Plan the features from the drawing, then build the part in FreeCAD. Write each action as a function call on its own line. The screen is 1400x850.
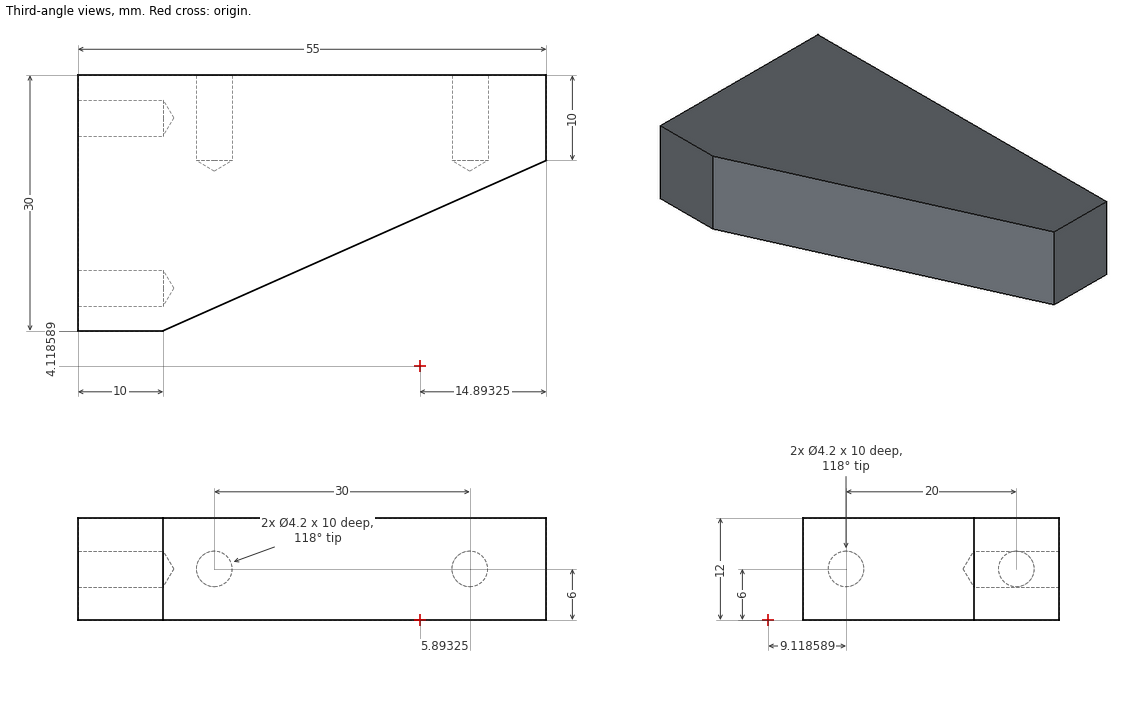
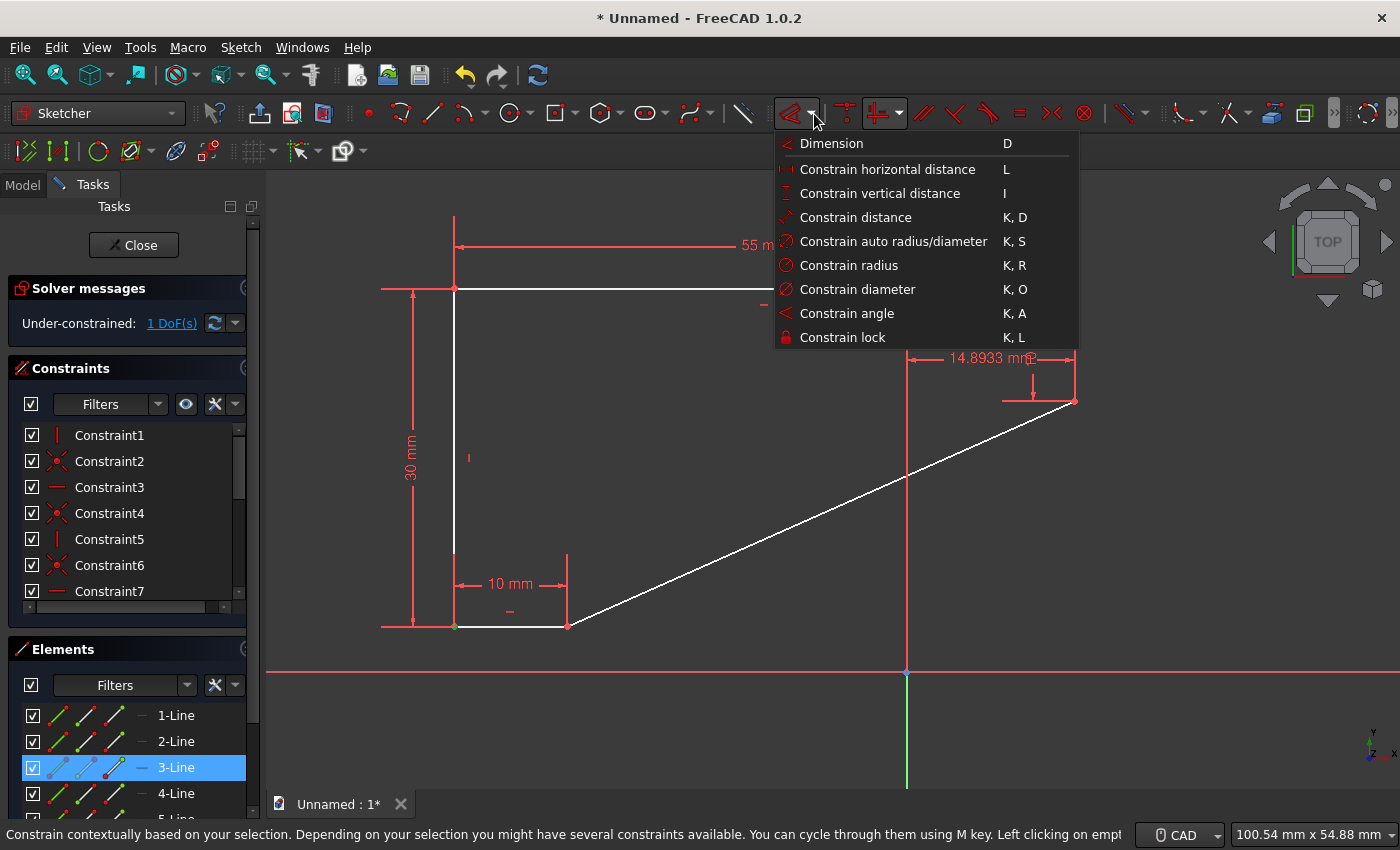
click(927, 193)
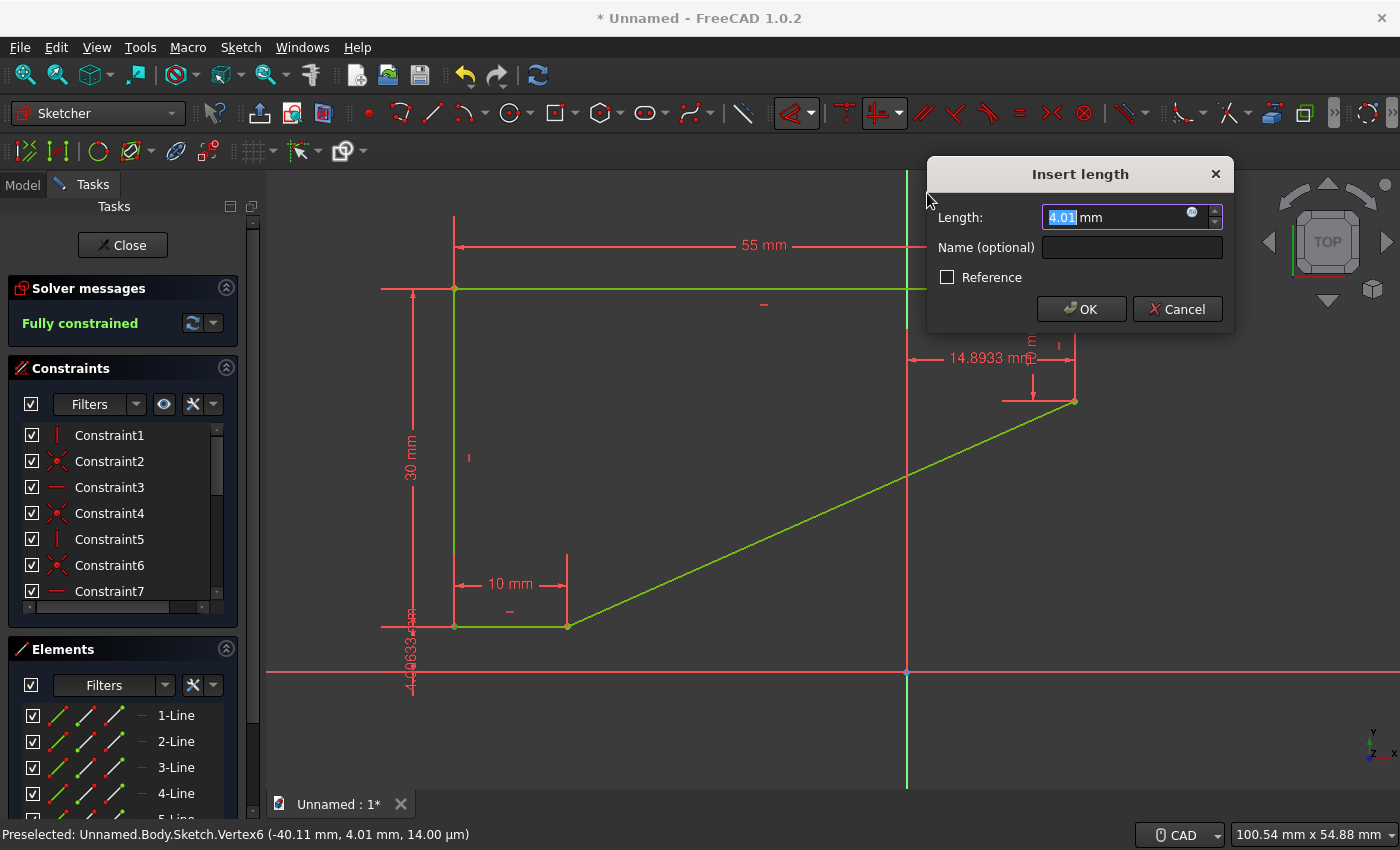
text(4.118589)
key(Return)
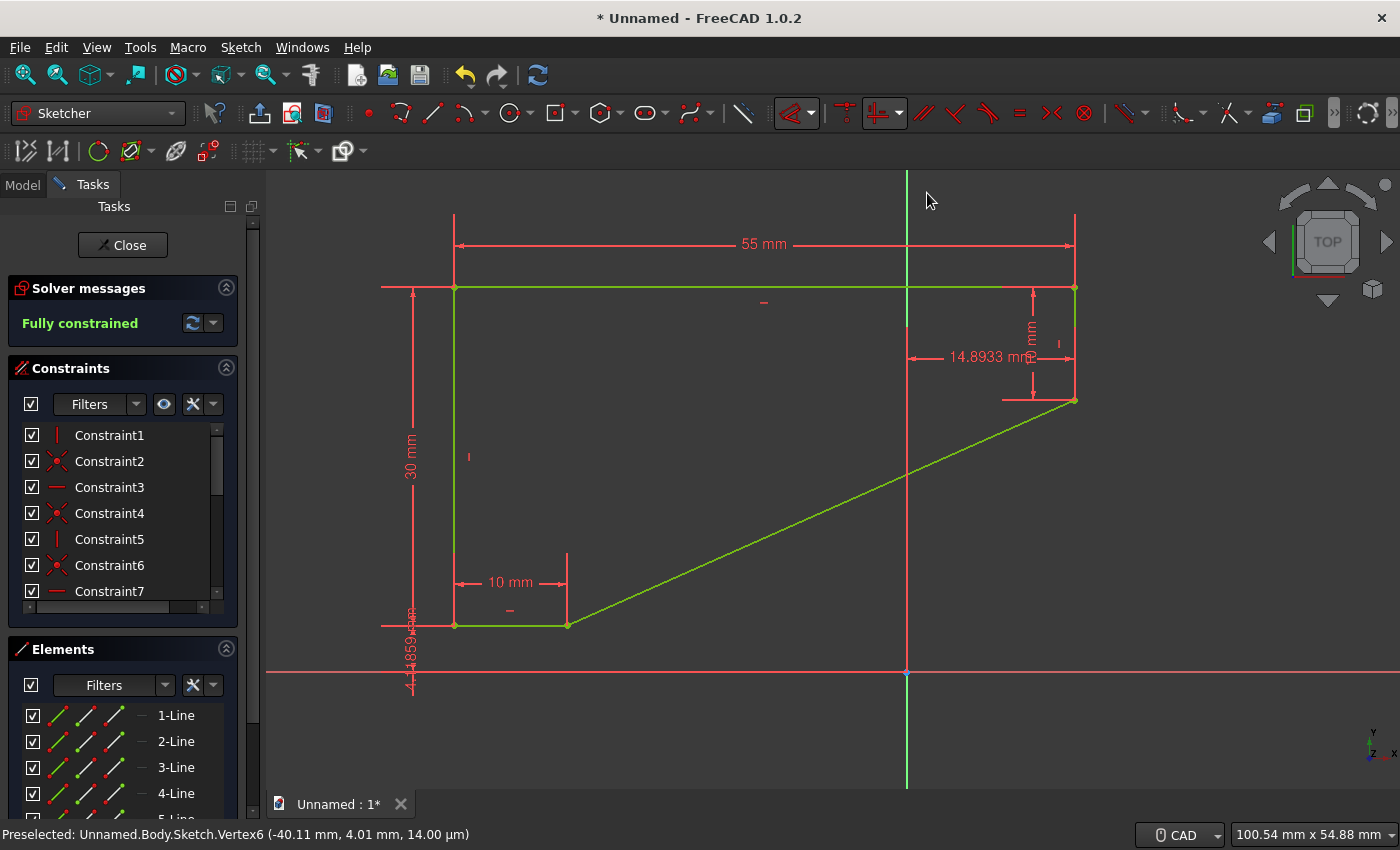
click(123, 245)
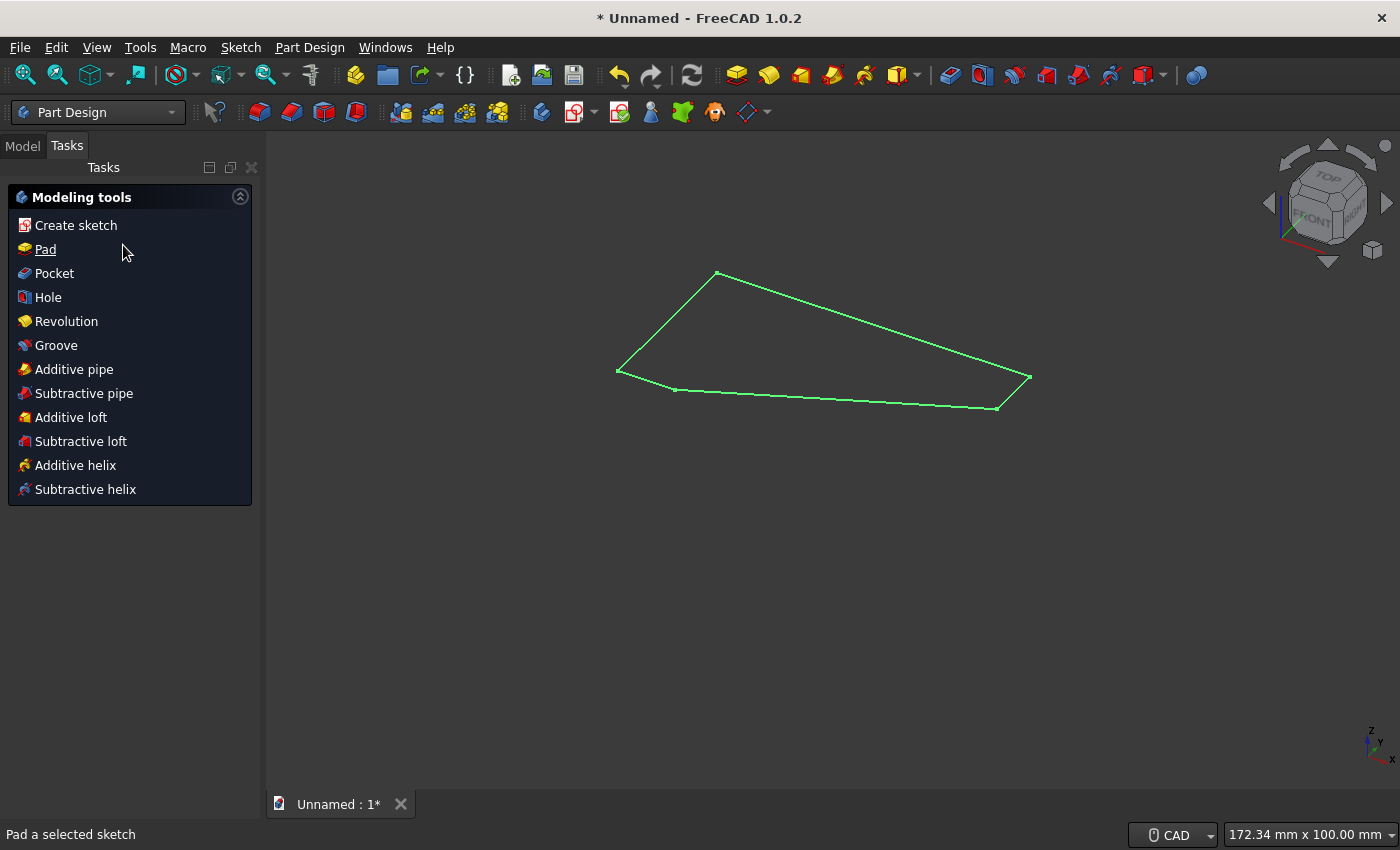
click(738, 76)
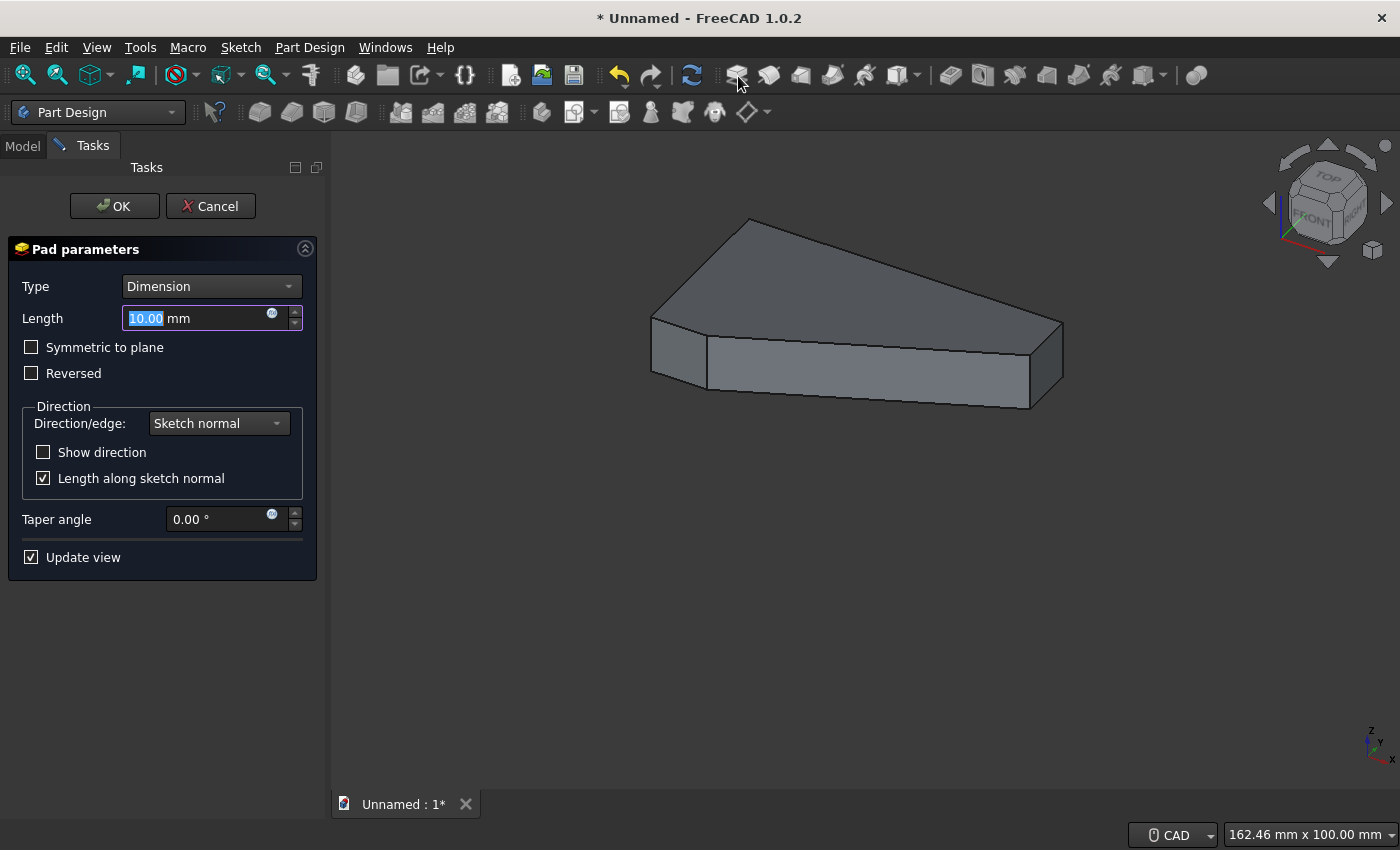
text(12)
key(Tab)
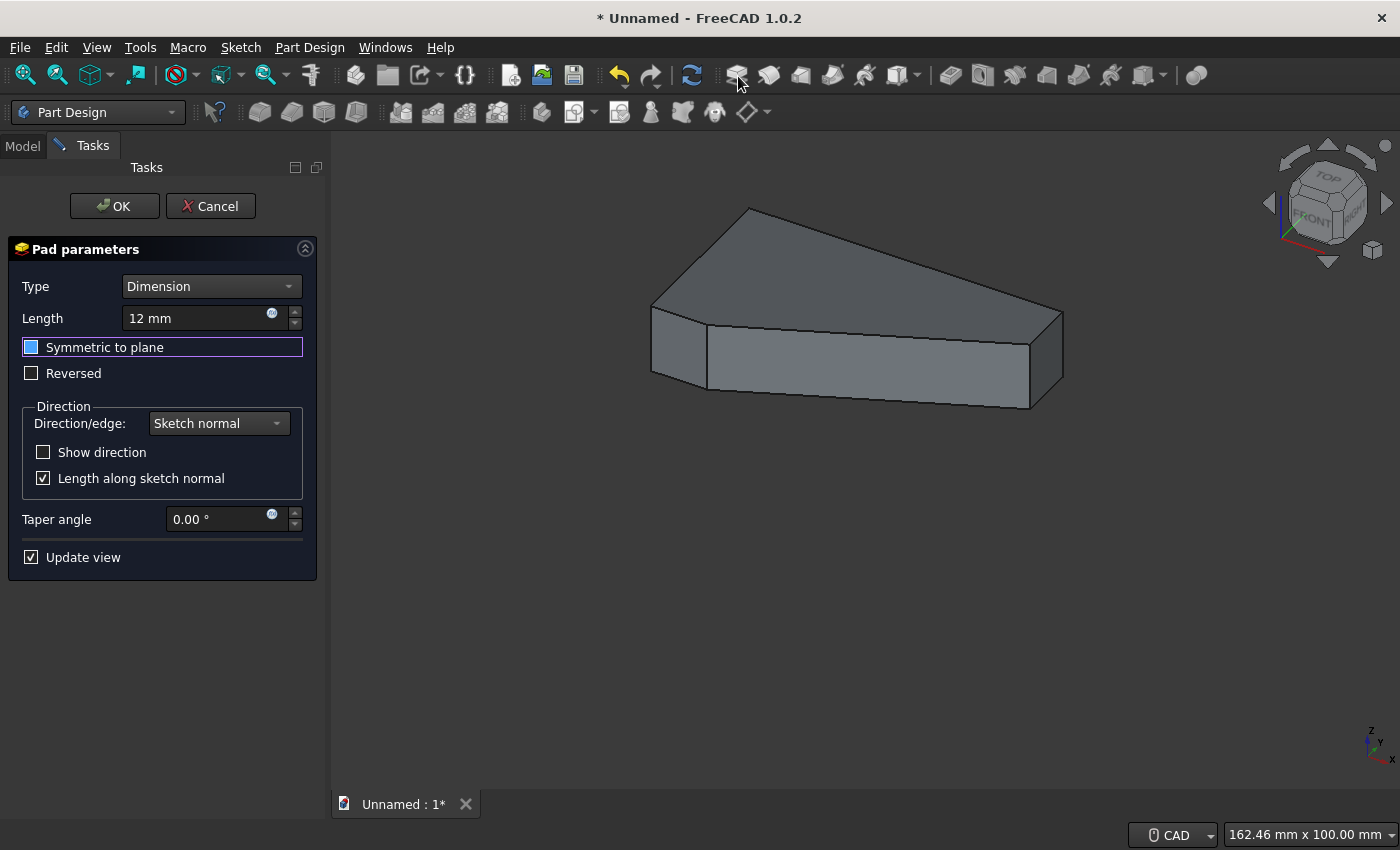
click(115, 206)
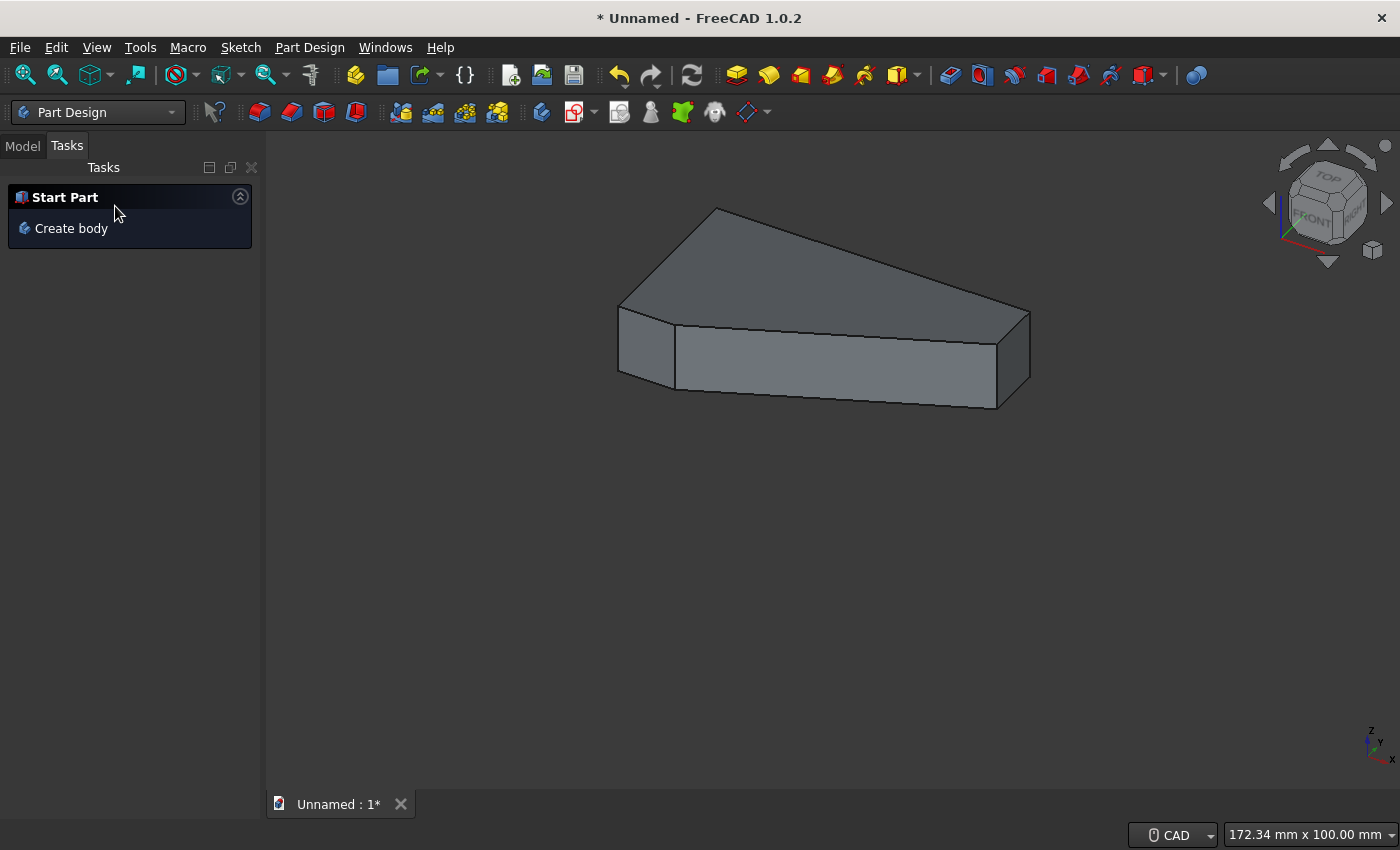
key(v)
key(f)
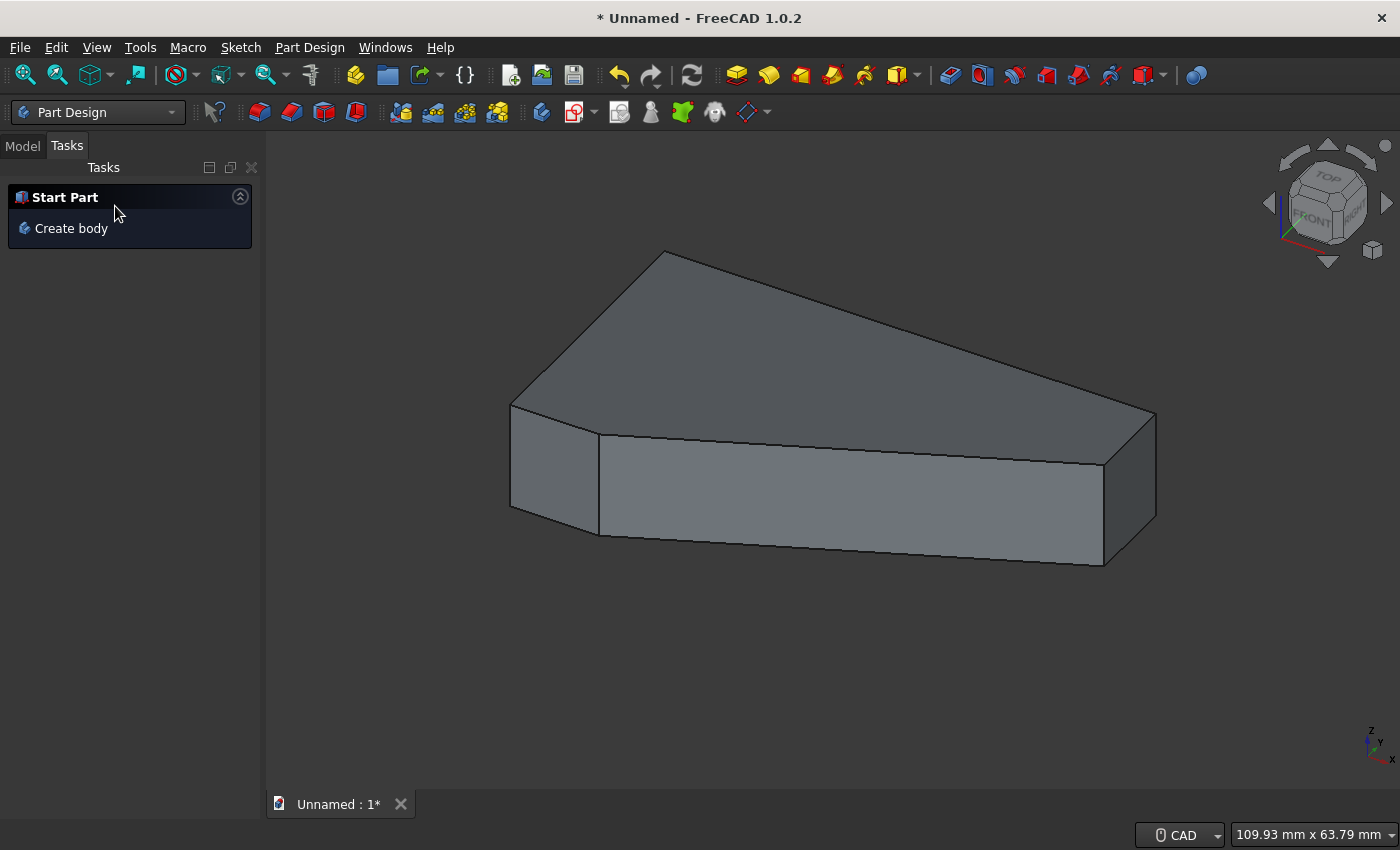
key(4)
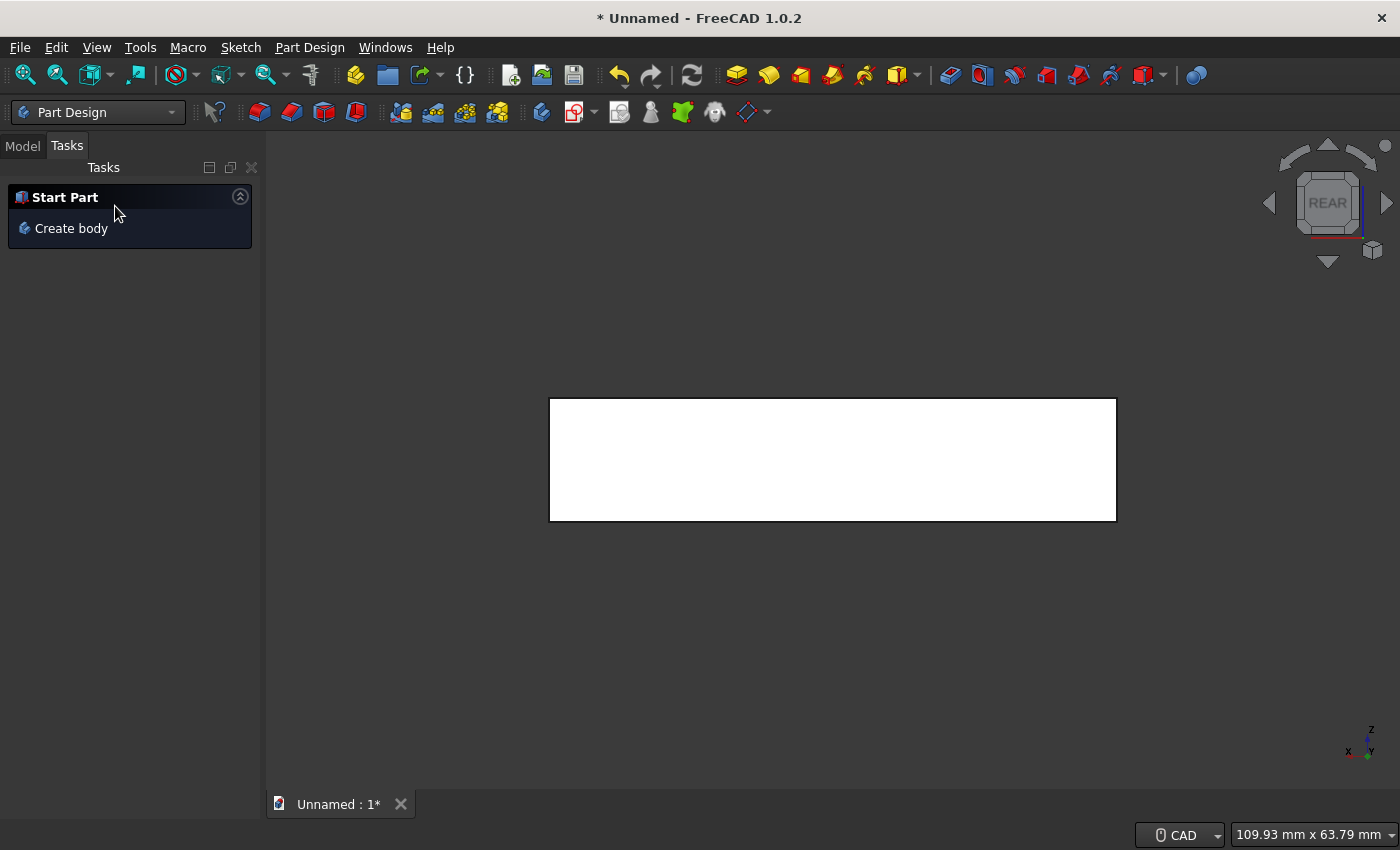
click(671, 459)